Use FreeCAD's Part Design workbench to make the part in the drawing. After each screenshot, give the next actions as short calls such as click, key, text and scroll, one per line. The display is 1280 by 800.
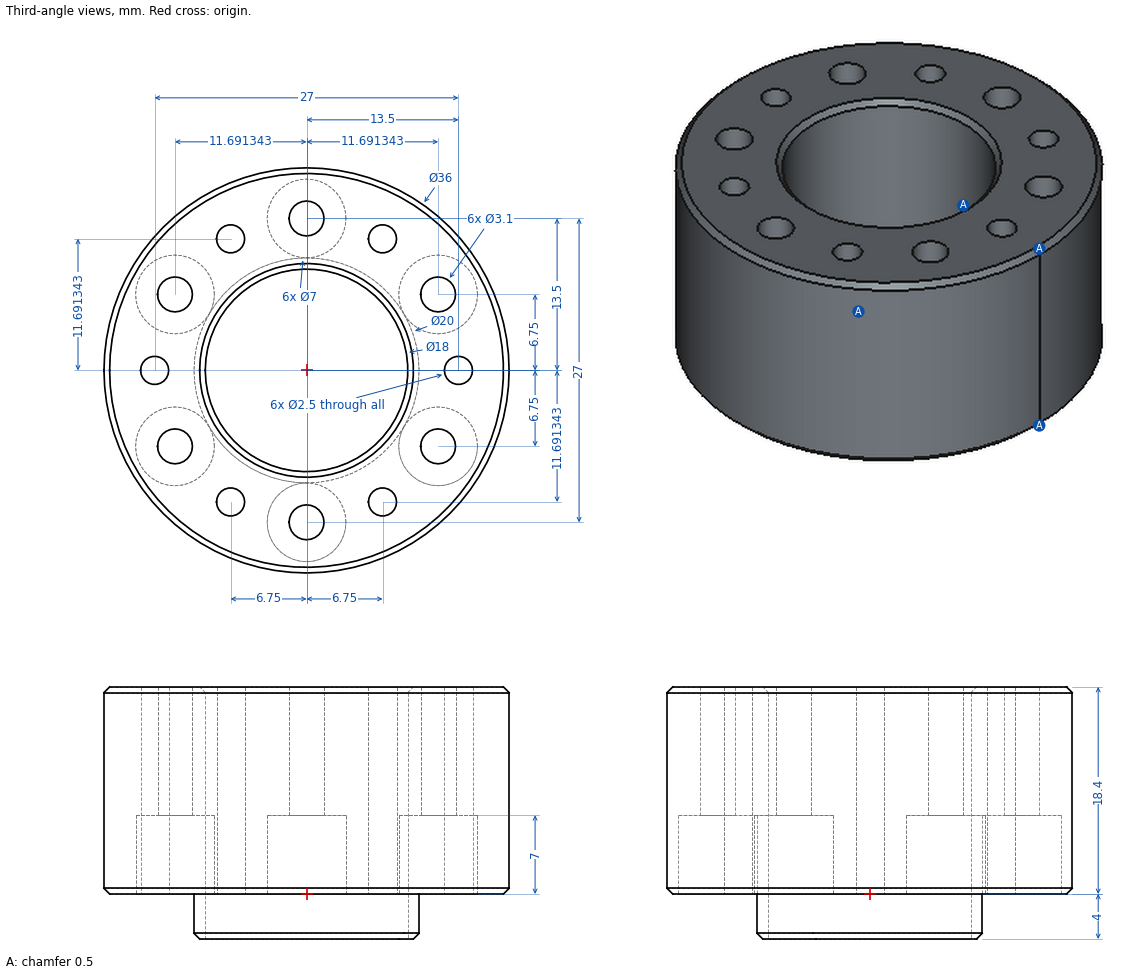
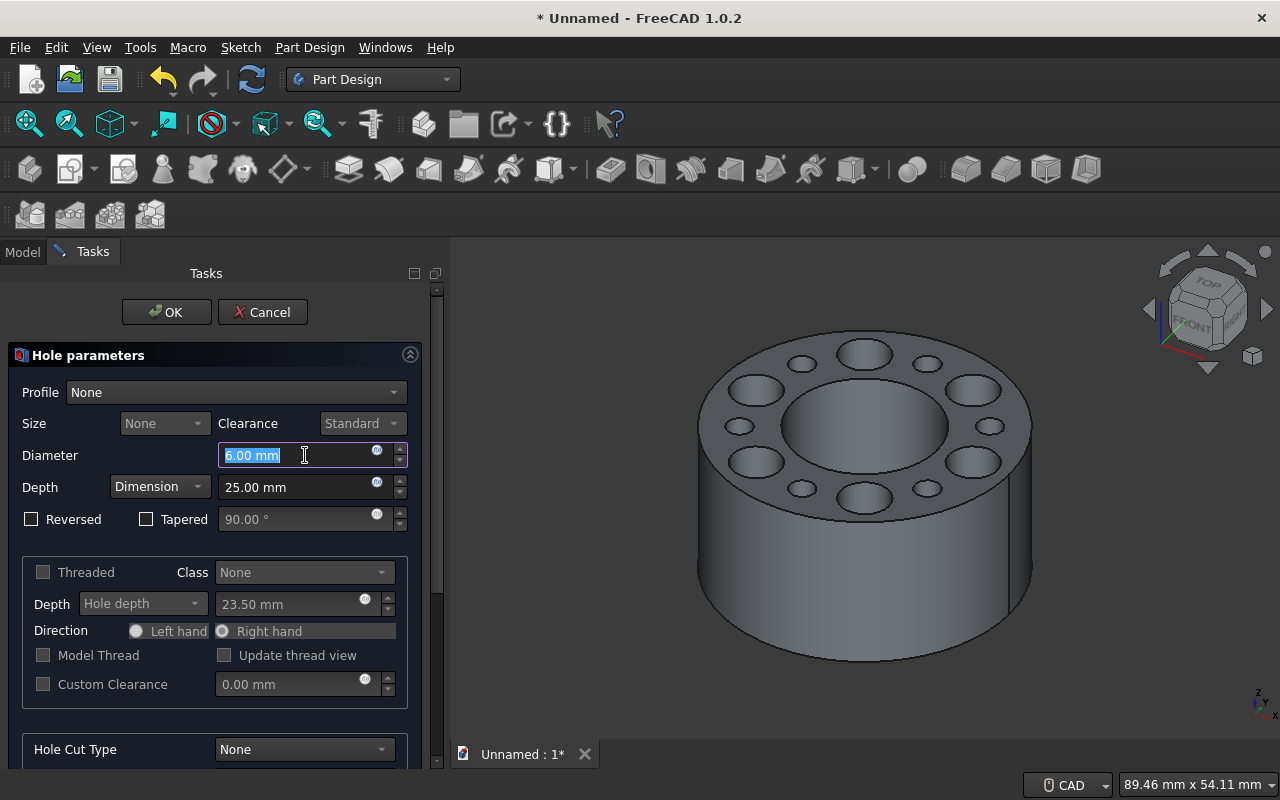
text(2.5)
key(Tab)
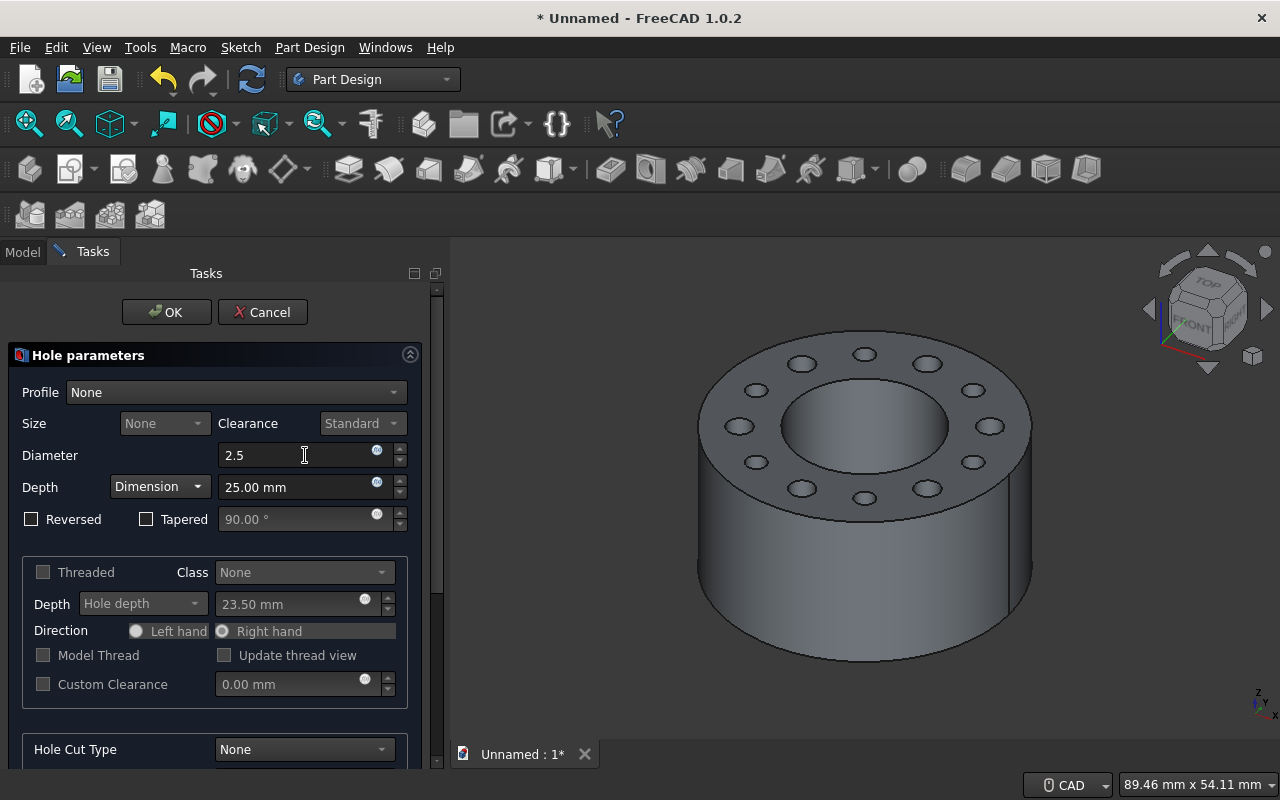
click(161, 486)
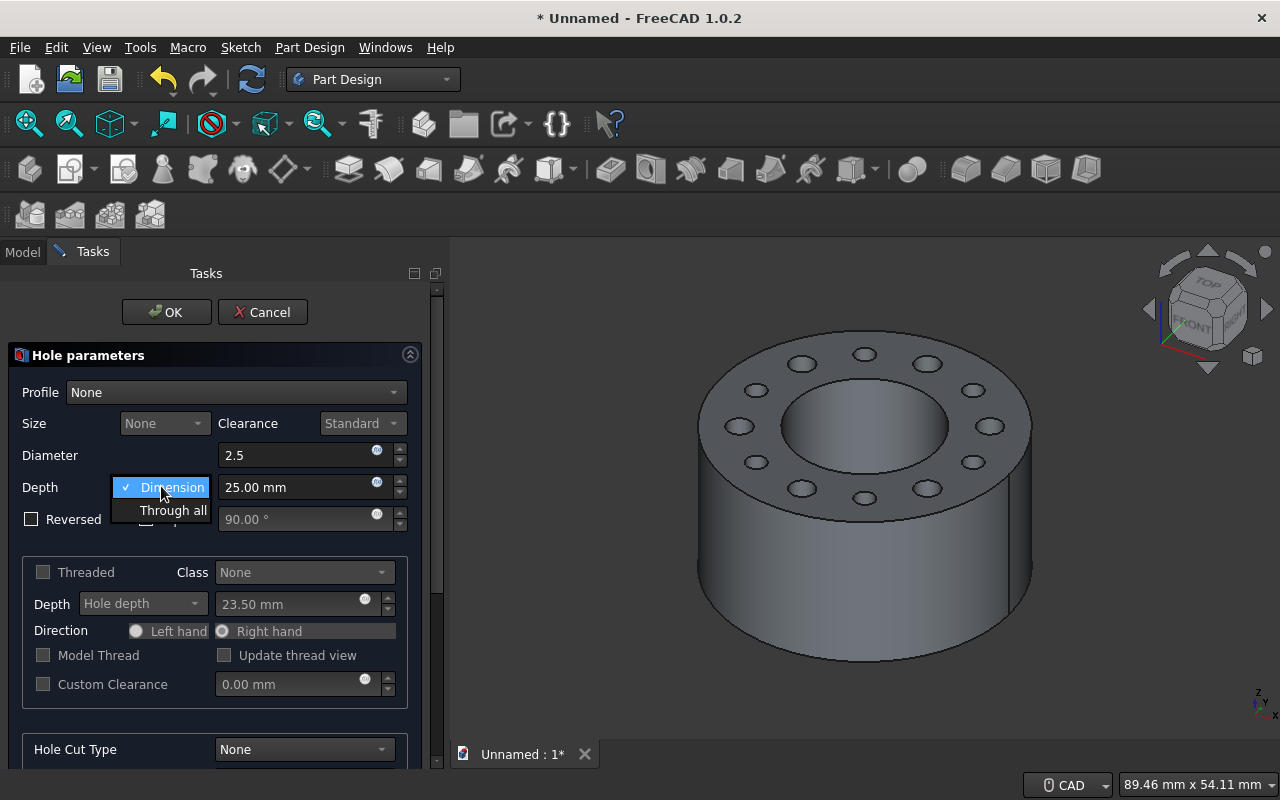
click(160, 510)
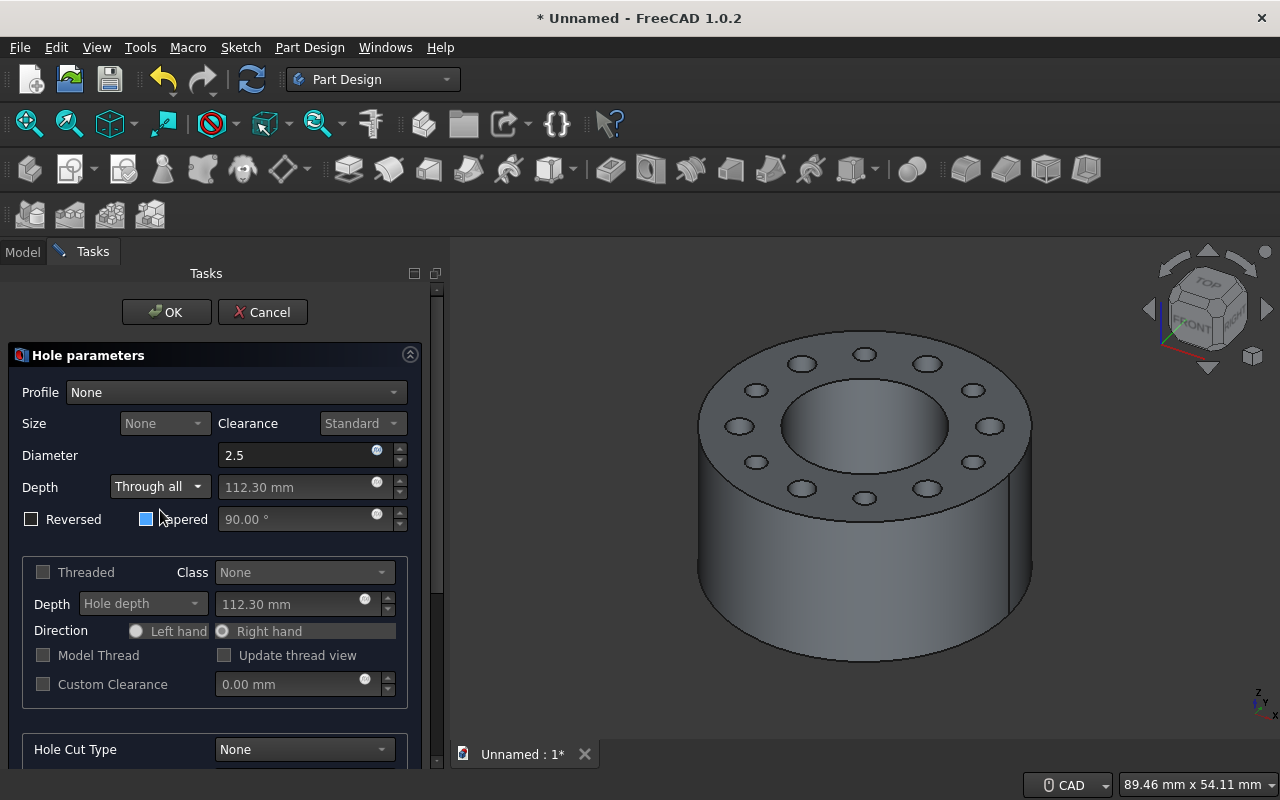
click(167, 312)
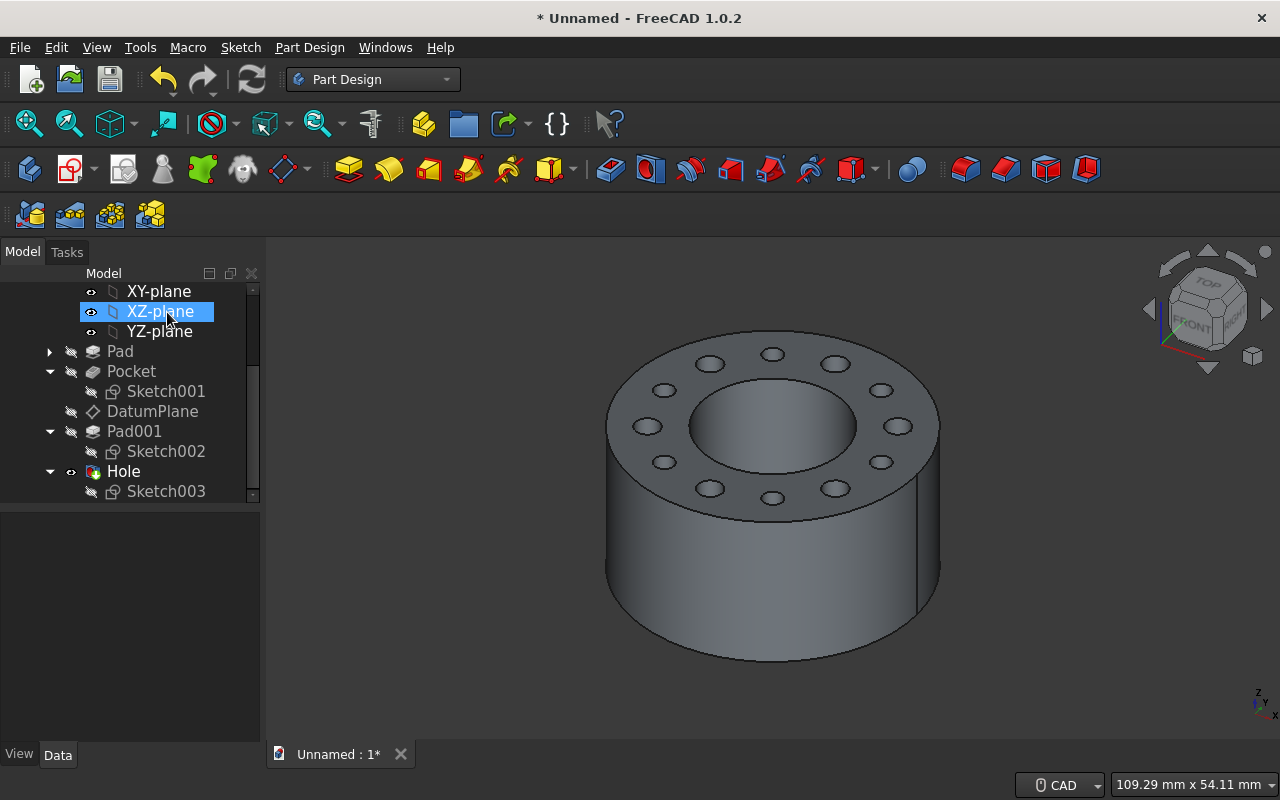
click(701, 401)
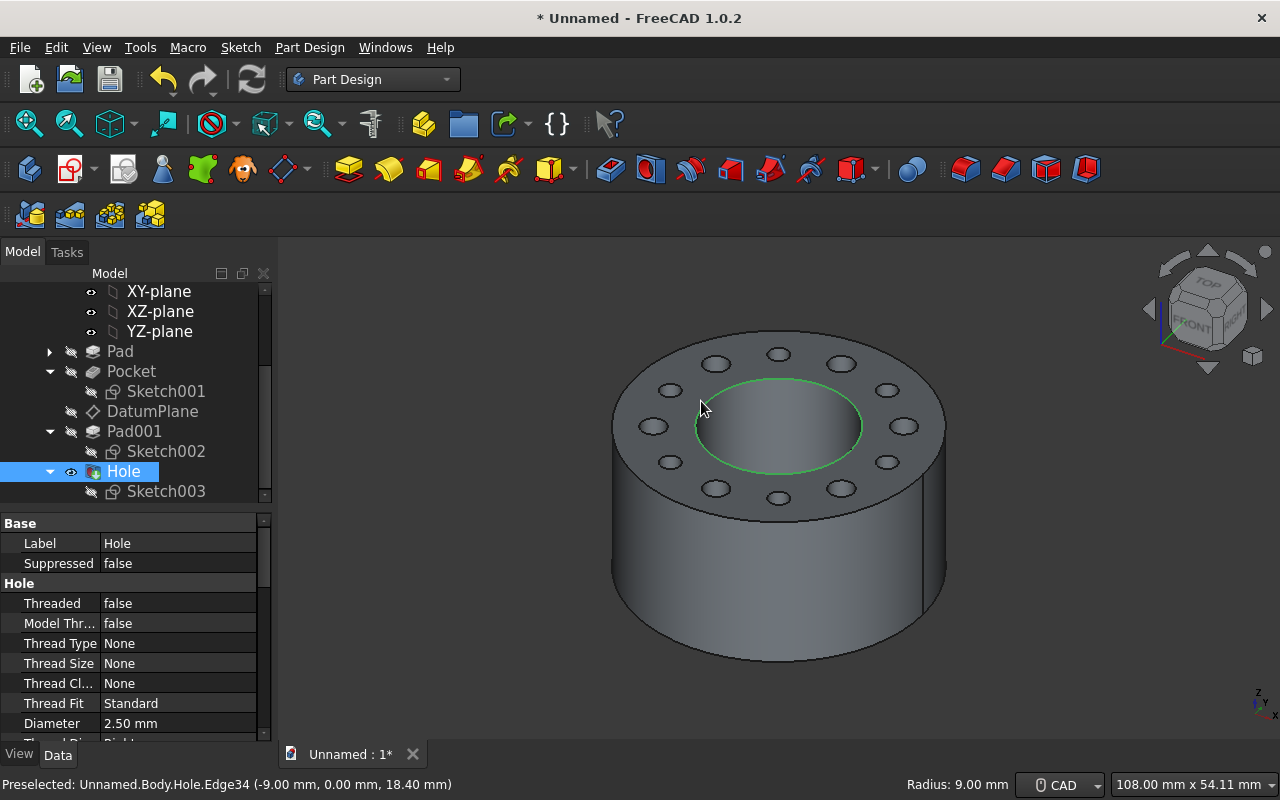
click(613, 435, ctrl)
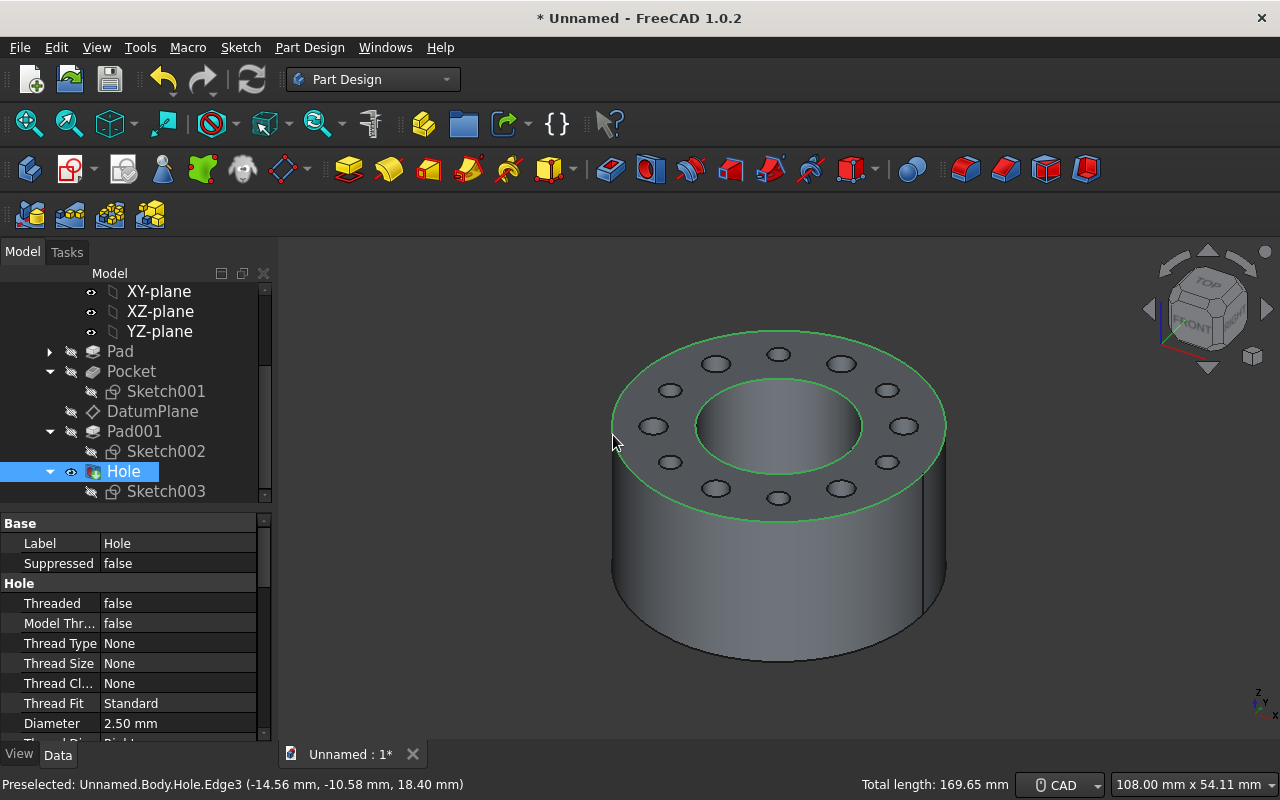
key(0)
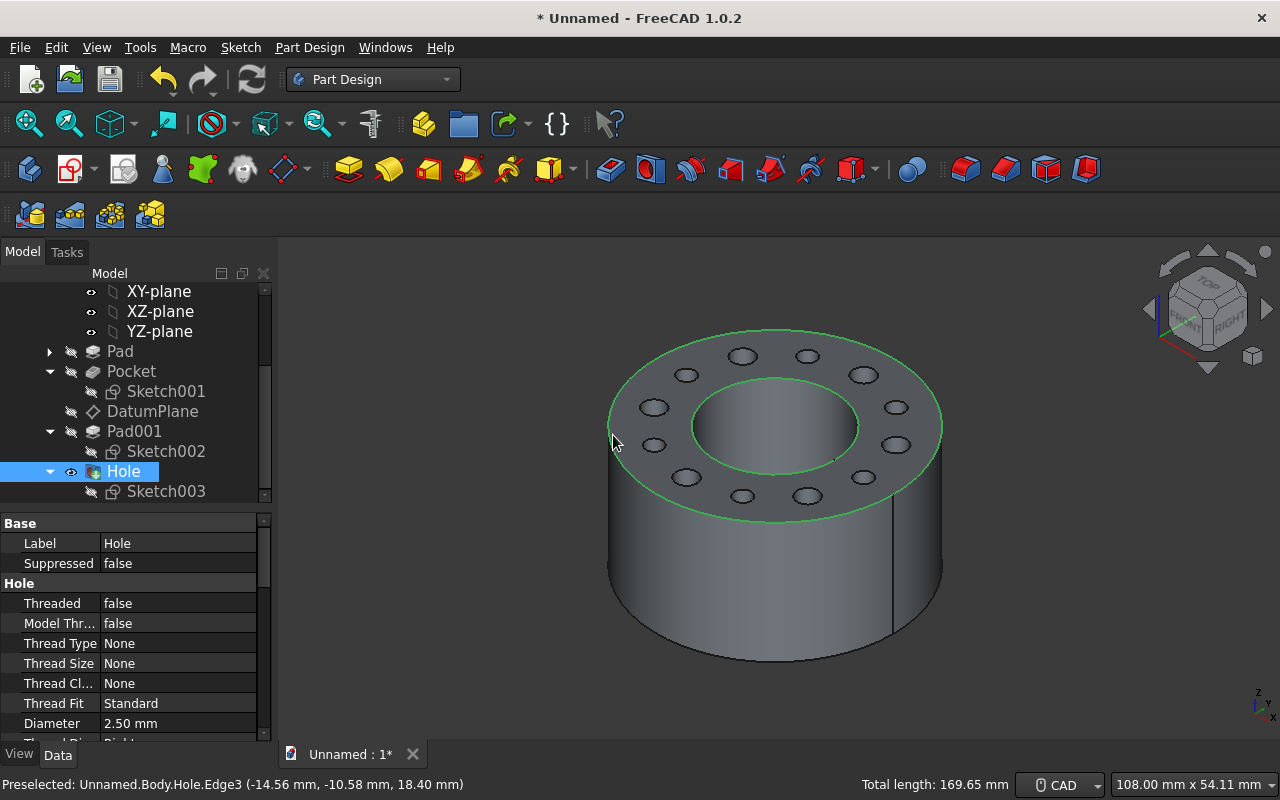
key(2)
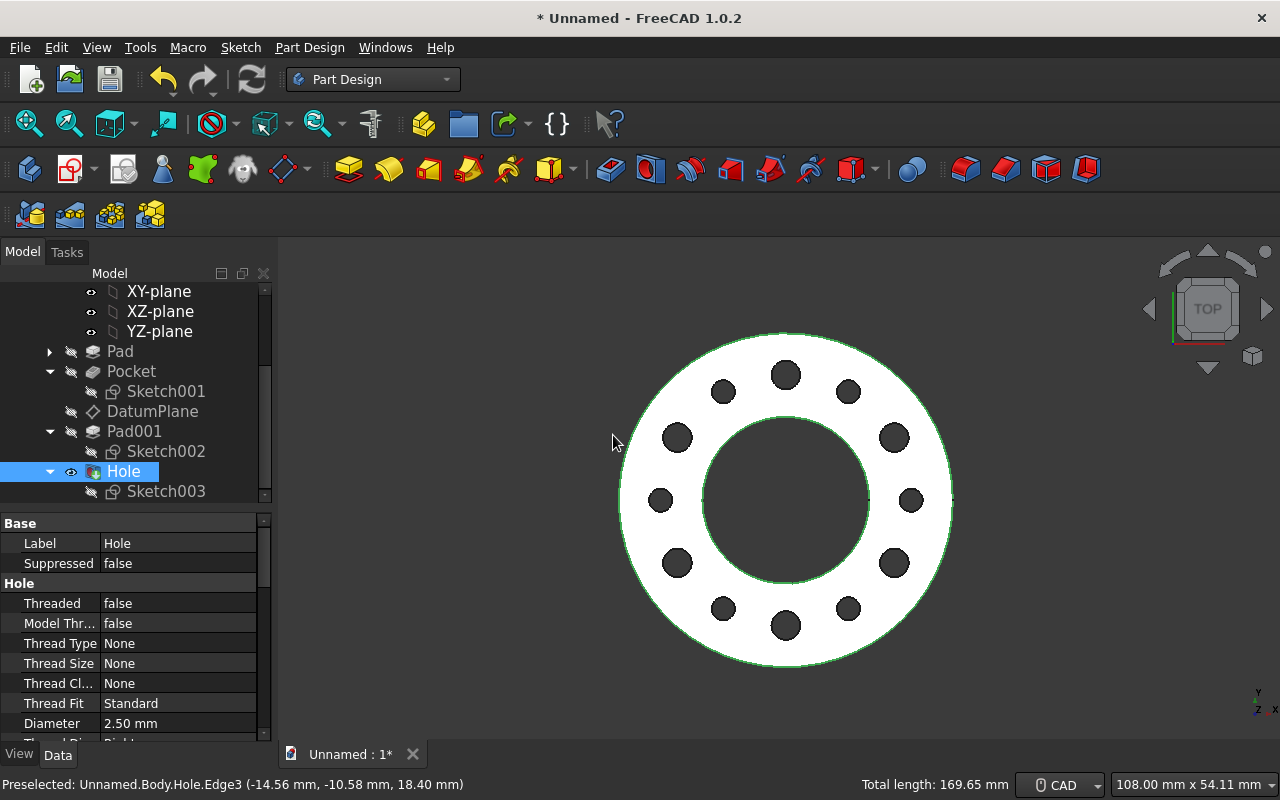
key(1)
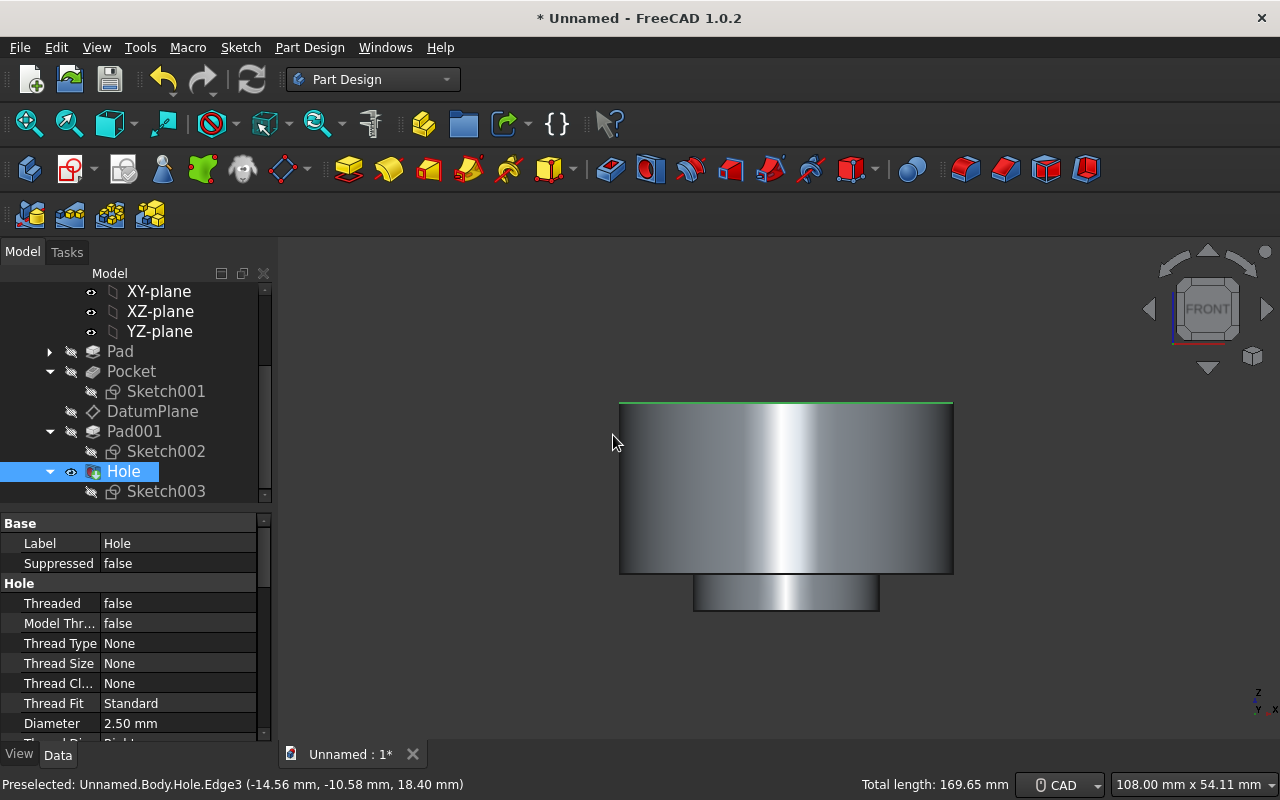
click(30, 124)